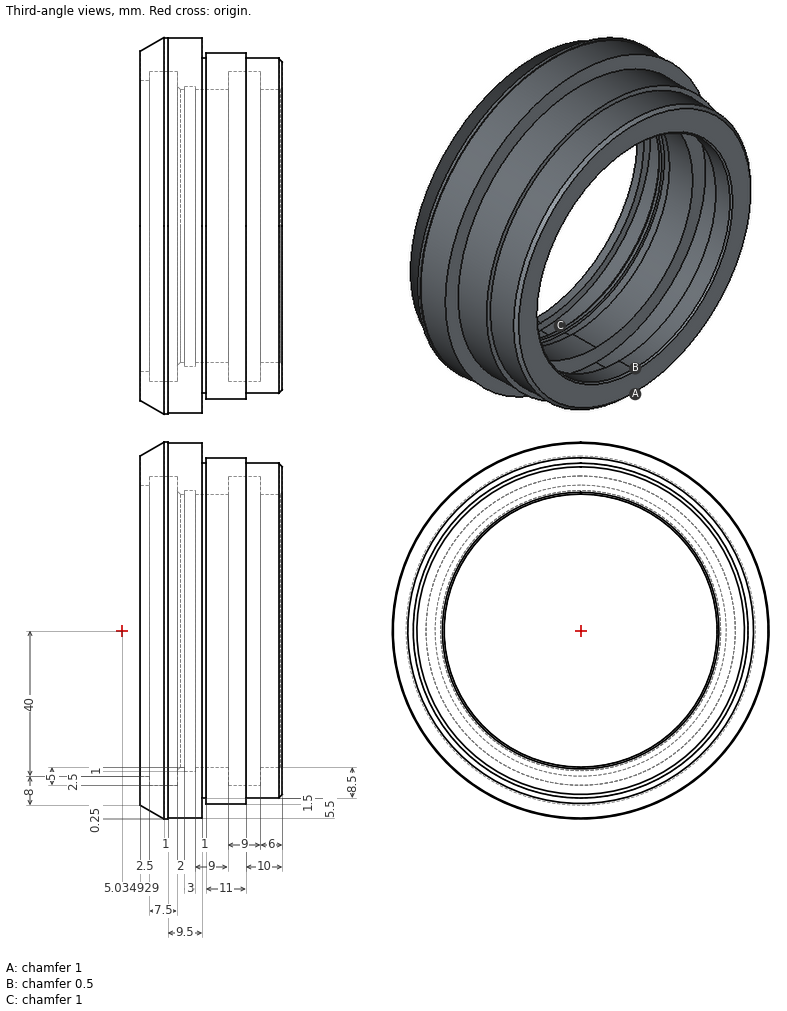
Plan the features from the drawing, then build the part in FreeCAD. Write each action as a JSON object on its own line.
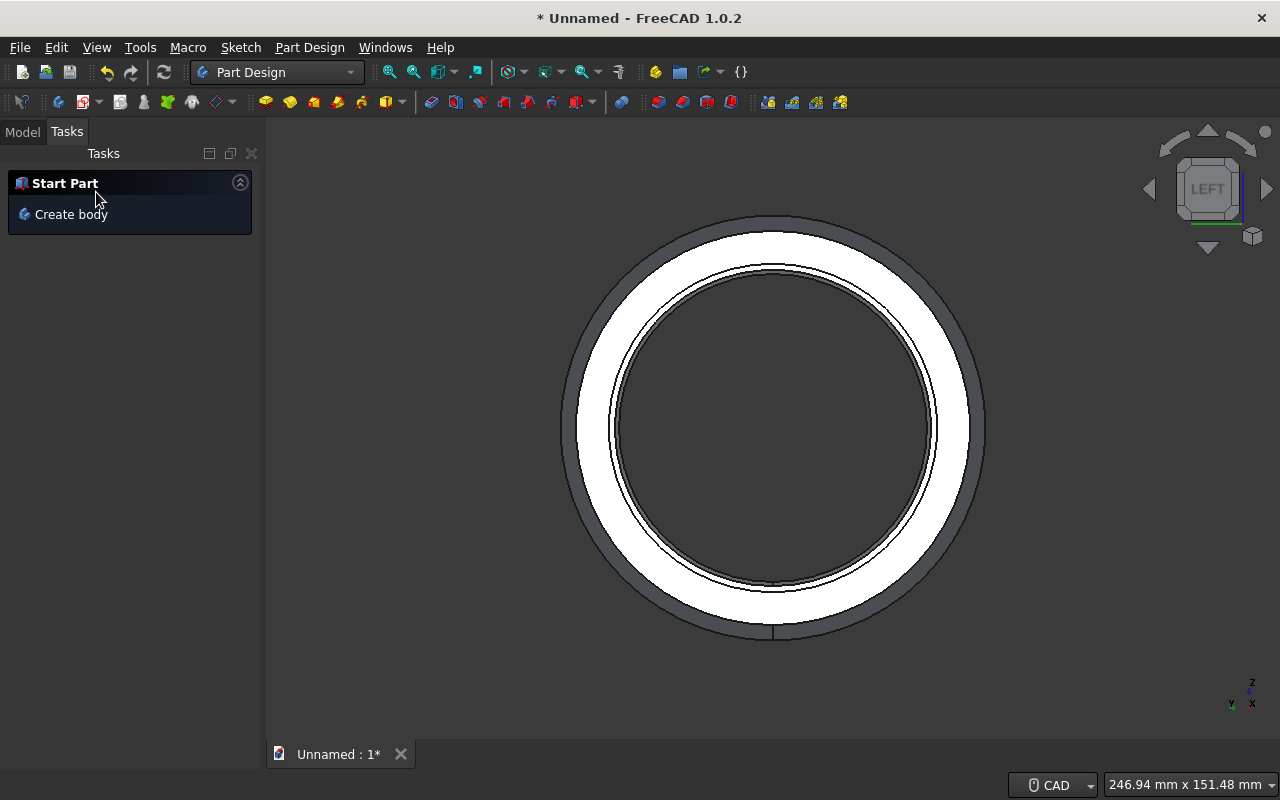
{"action": "key", "text": "0"}